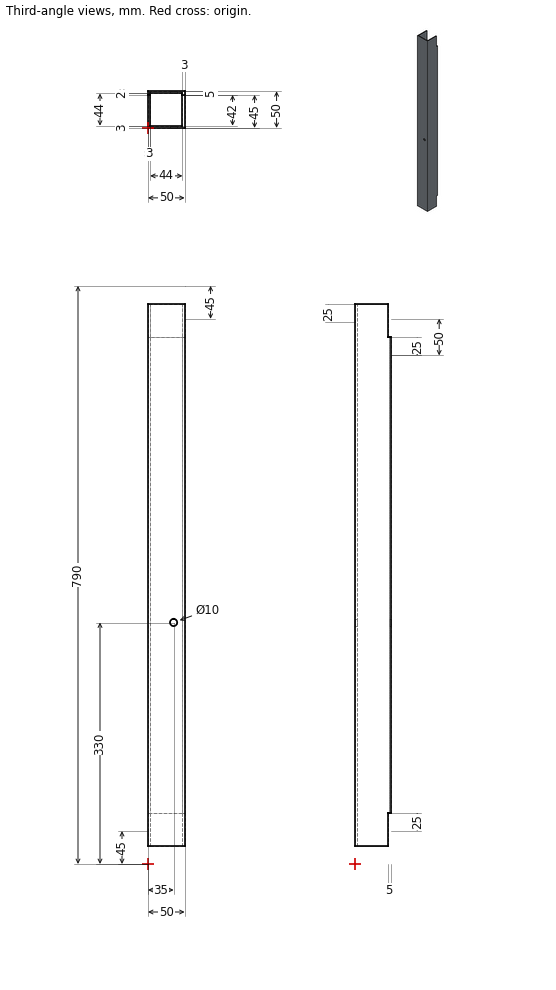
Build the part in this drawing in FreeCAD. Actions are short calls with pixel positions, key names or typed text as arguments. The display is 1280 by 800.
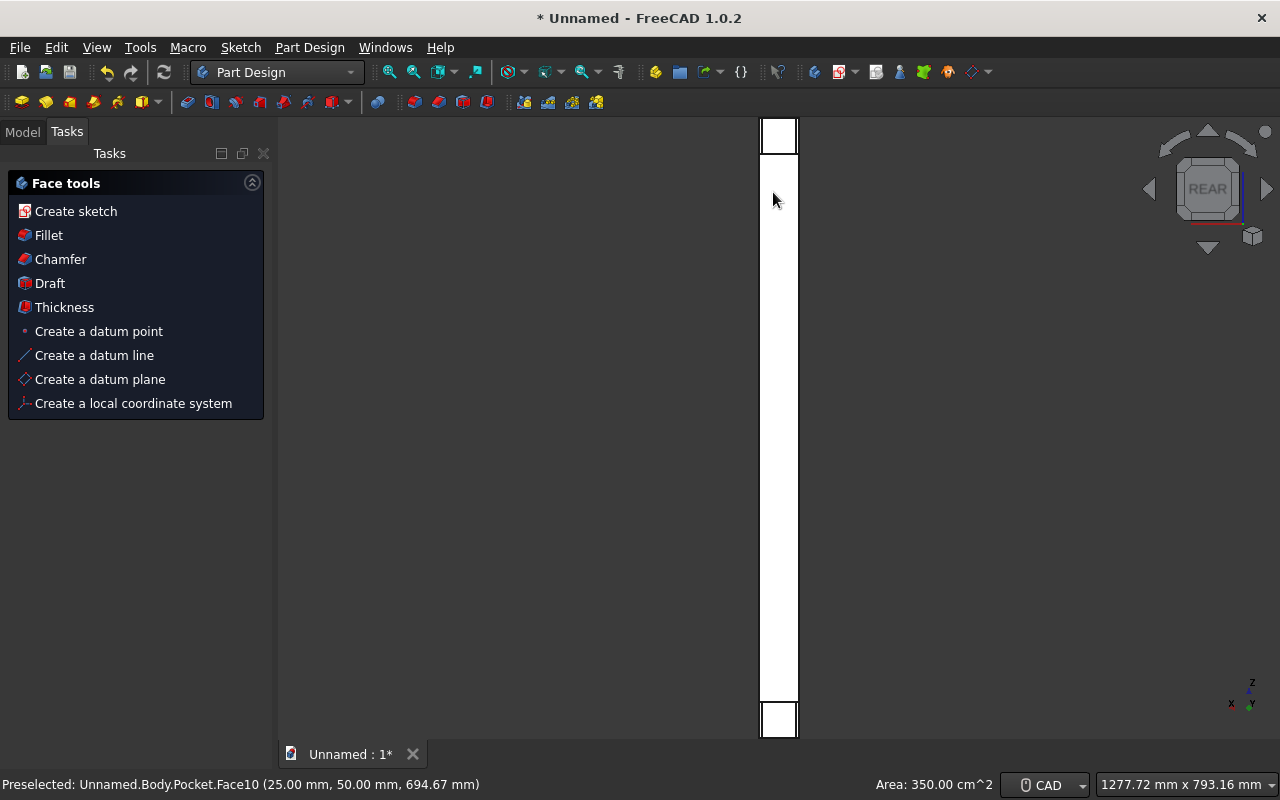
click(840, 72)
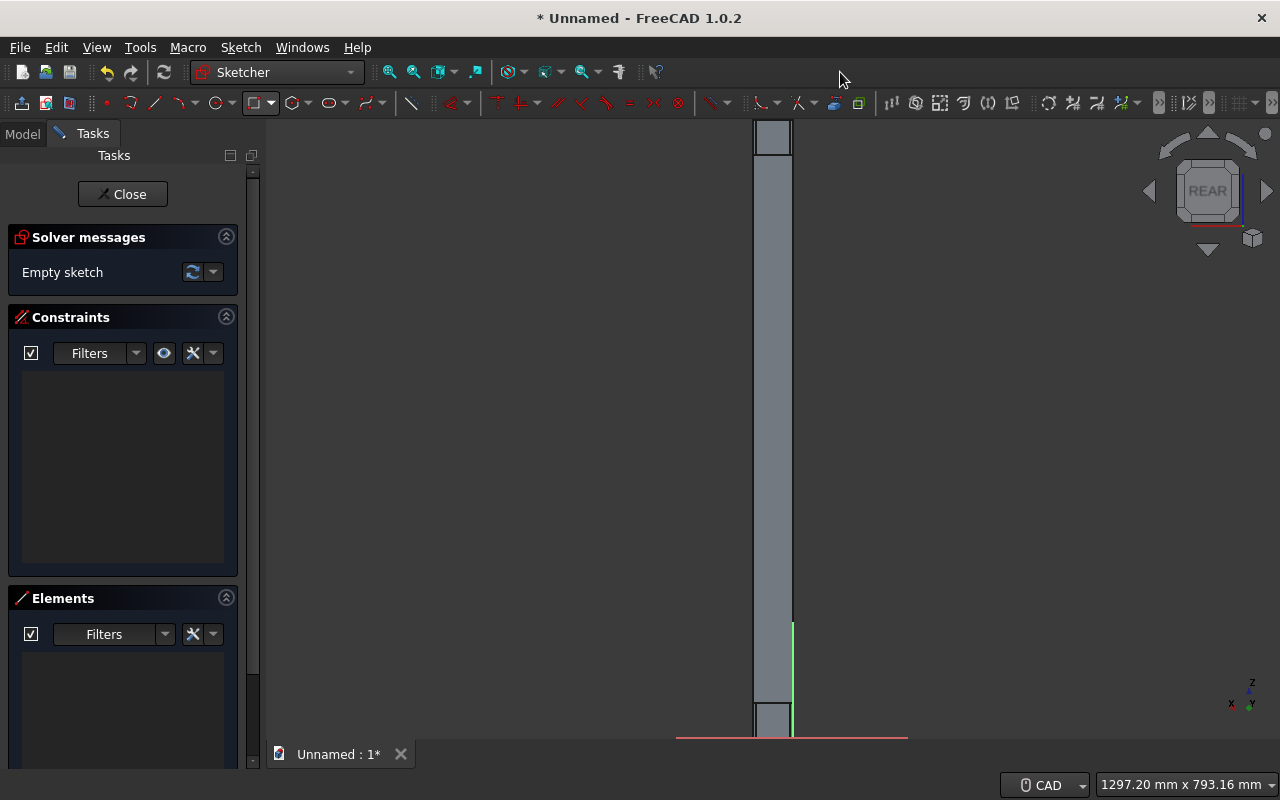
scroll(768, 482, up, 15)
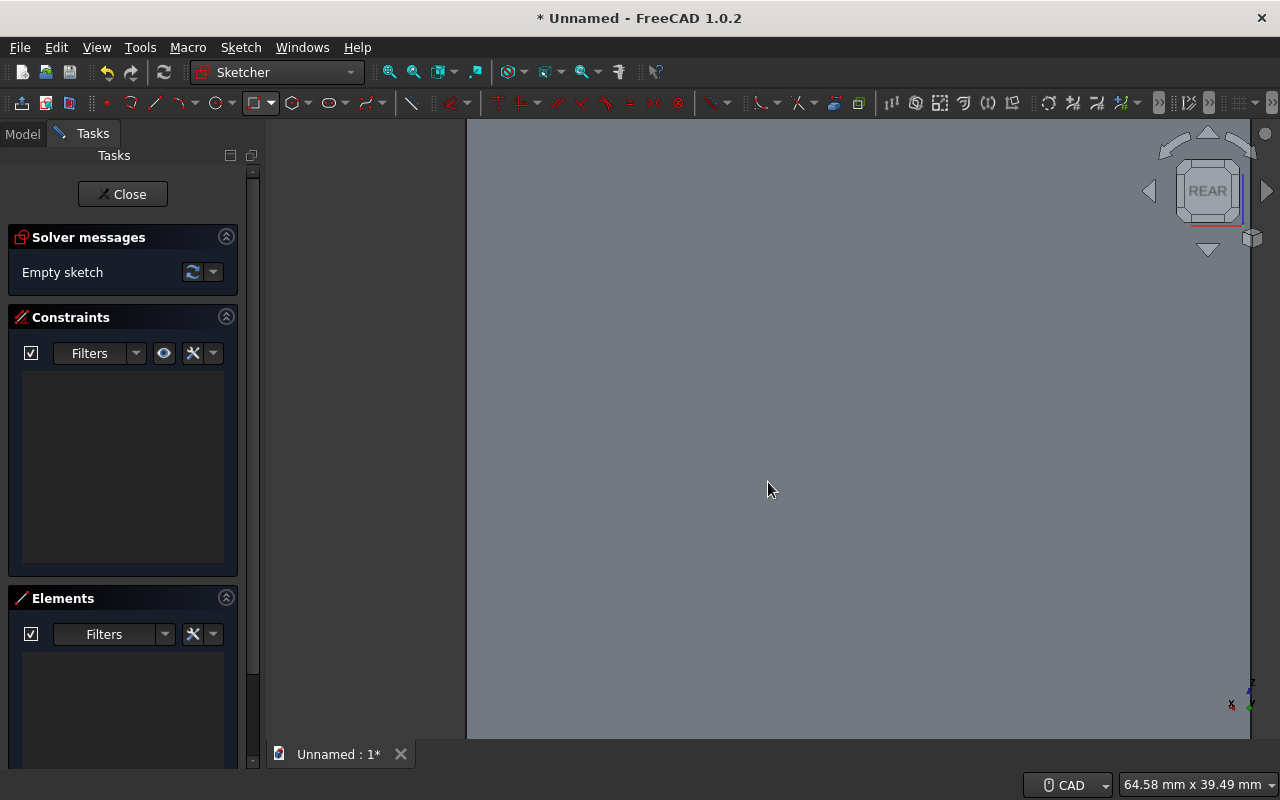
scroll(700, 426, up, 5)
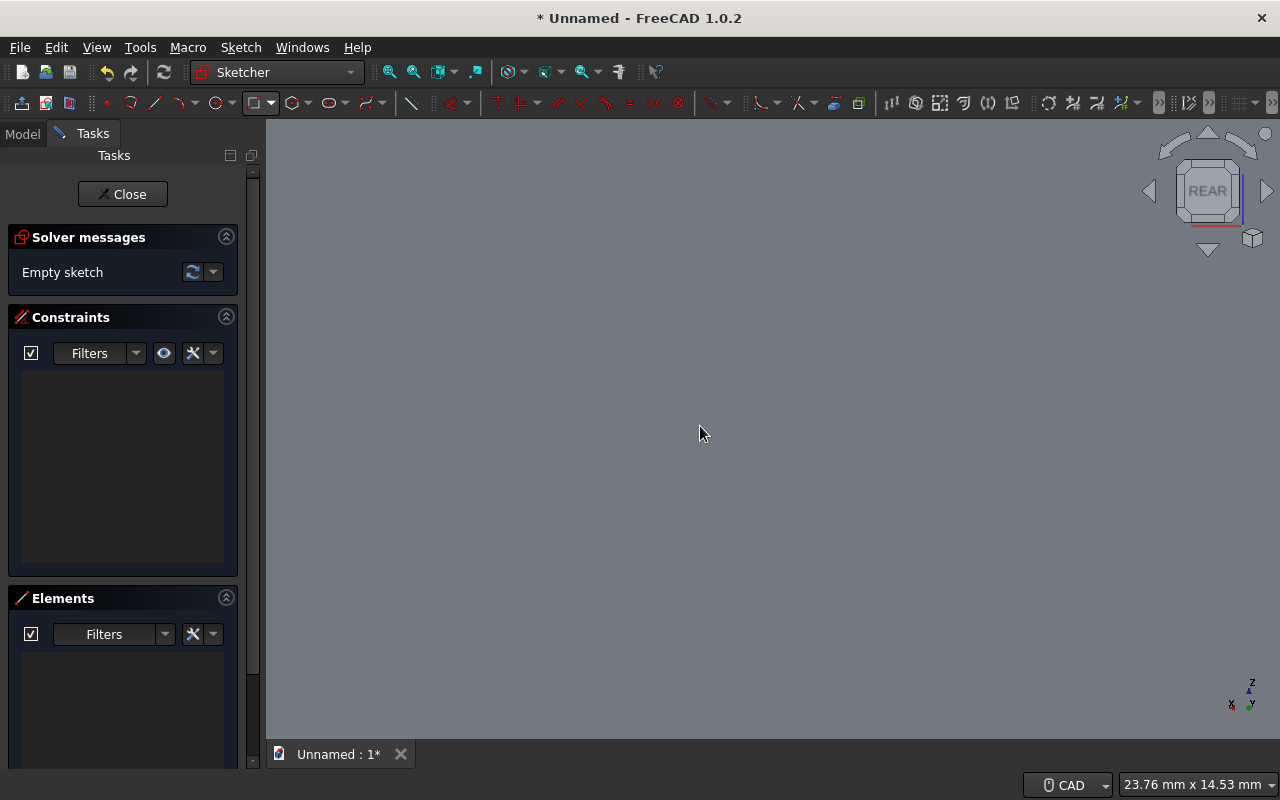
click(216, 104)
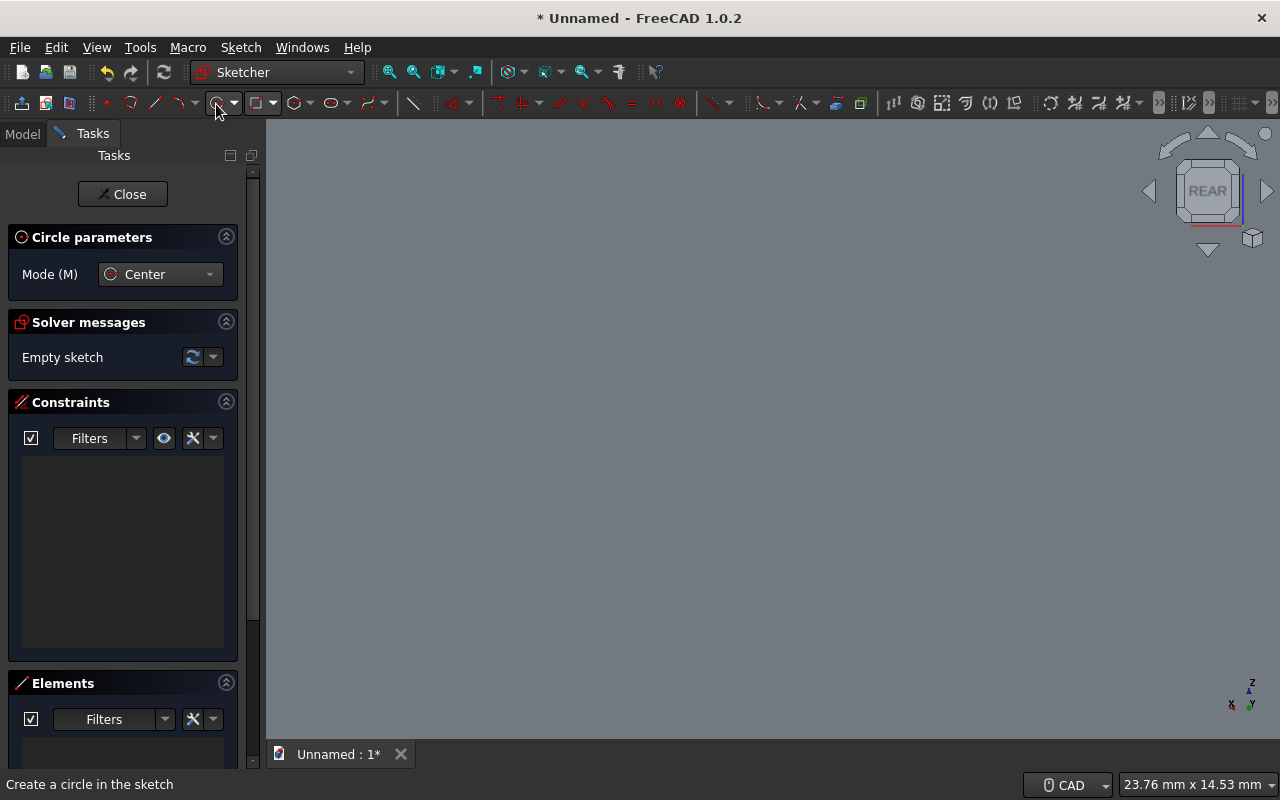
click(705, 427)
click(855, 276)
key(Escape)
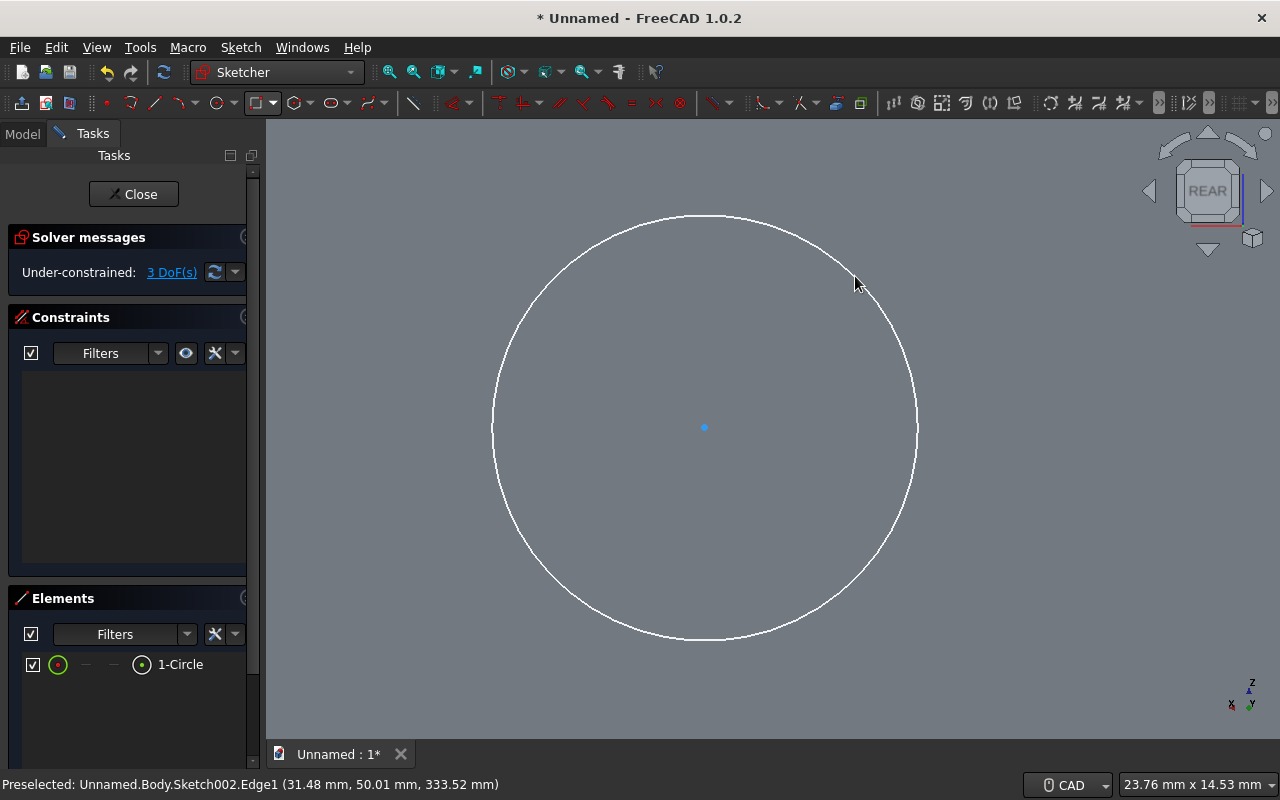
click(452, 104)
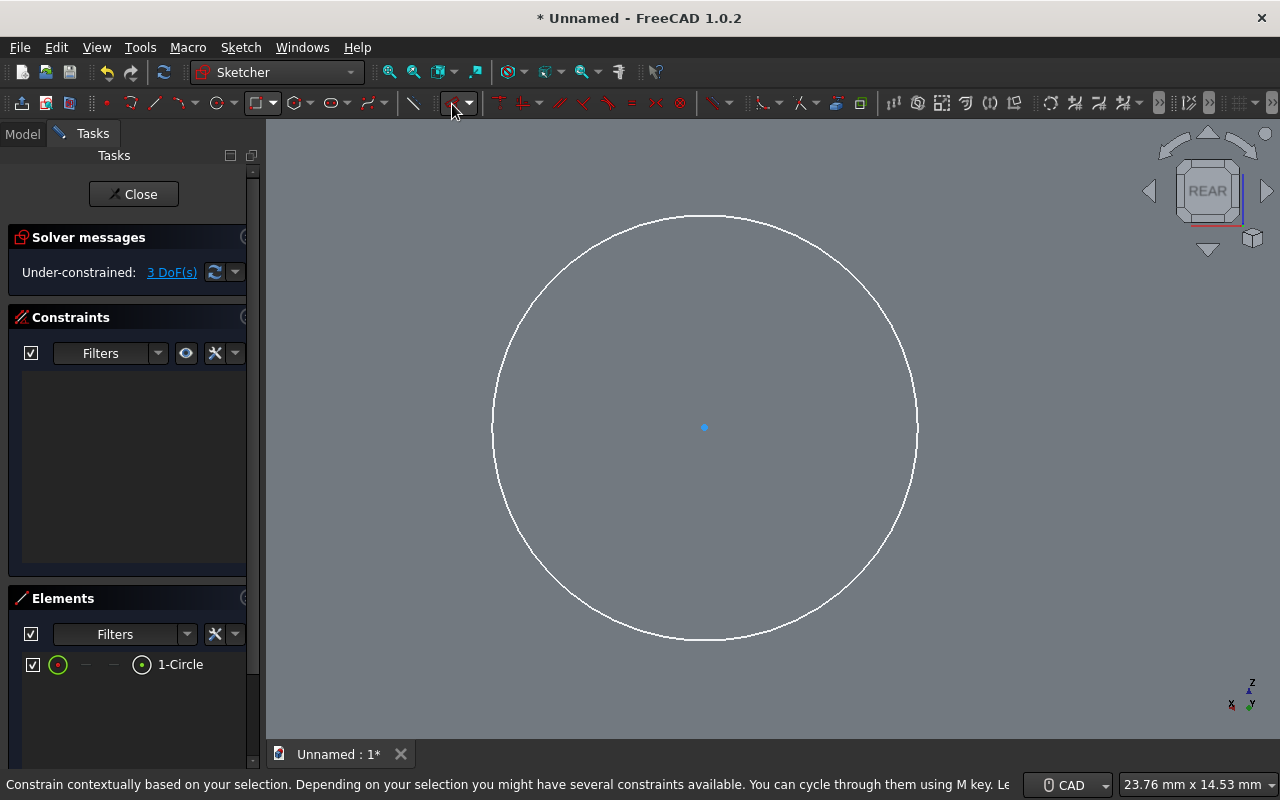
click(855, 277)
click(878, 254)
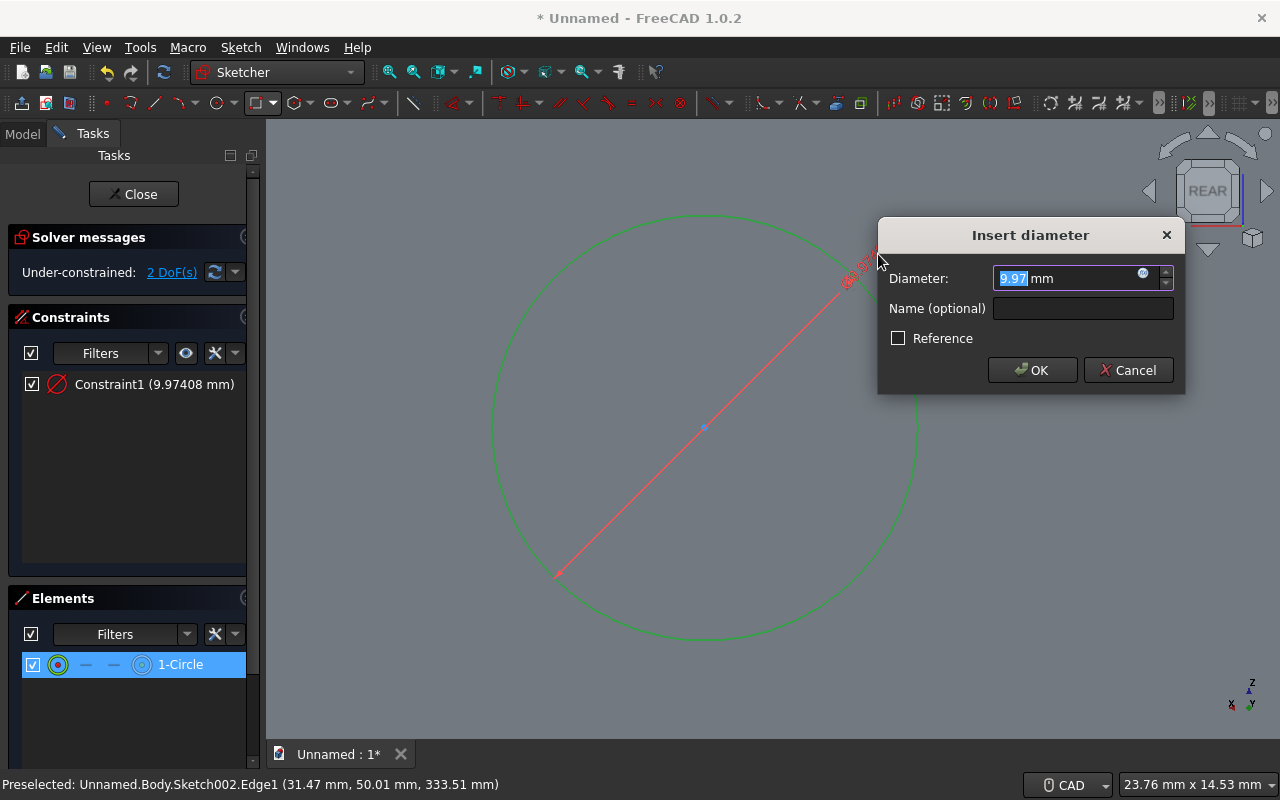
text(10)
key(Return)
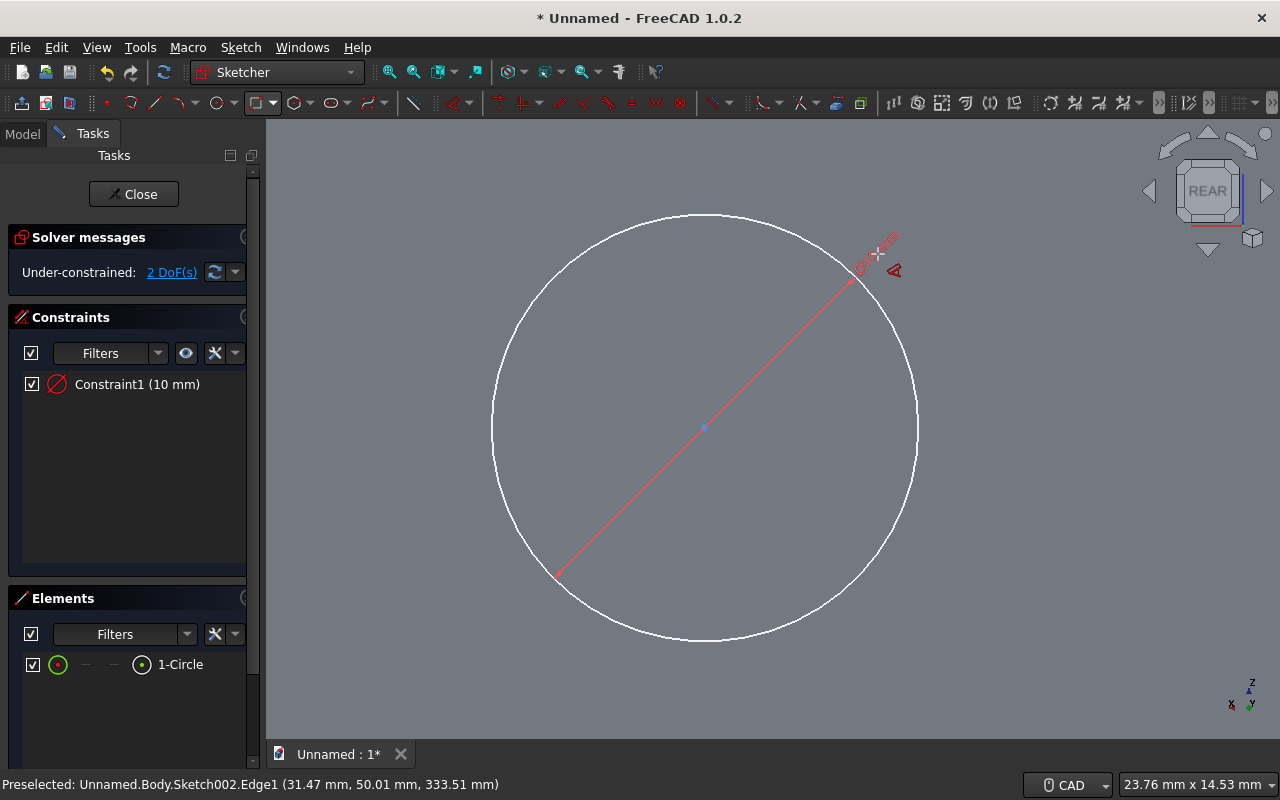
click(705, 428)
click(816, 394)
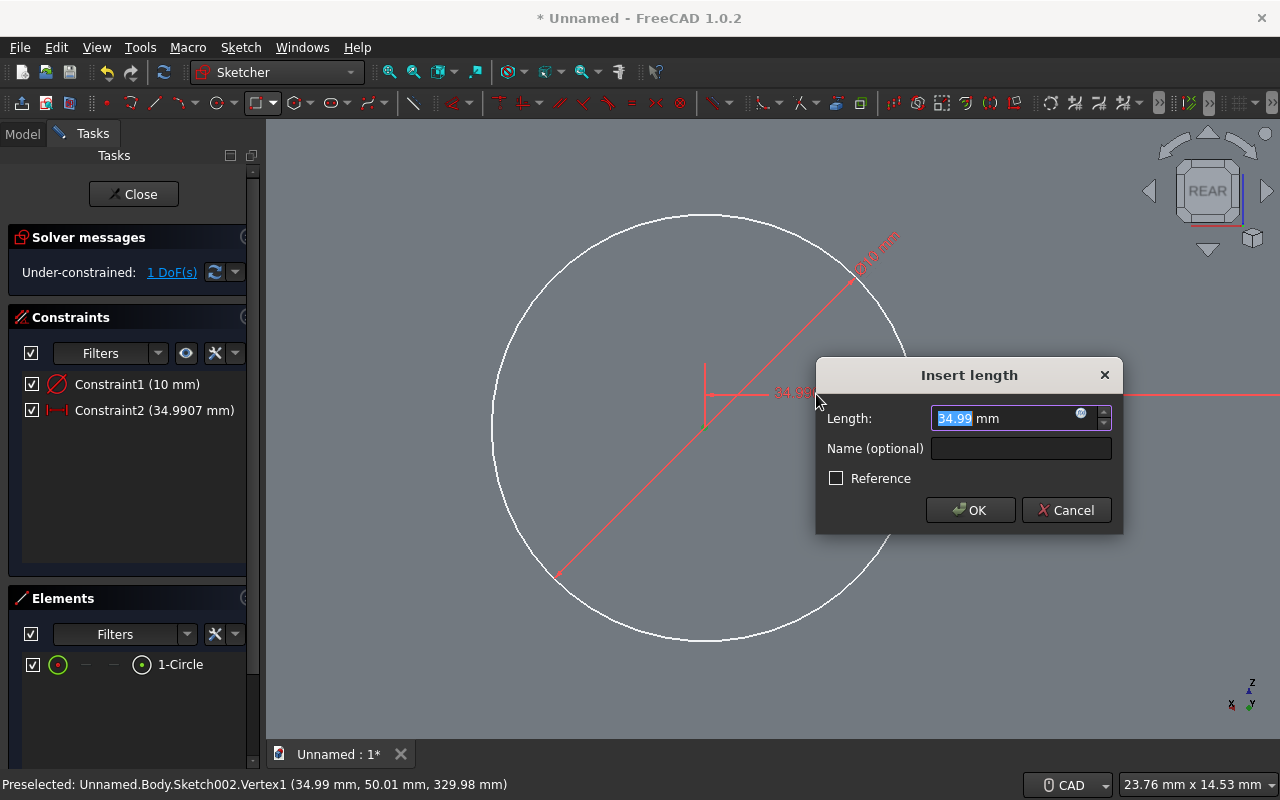
text(35)
key(Return)